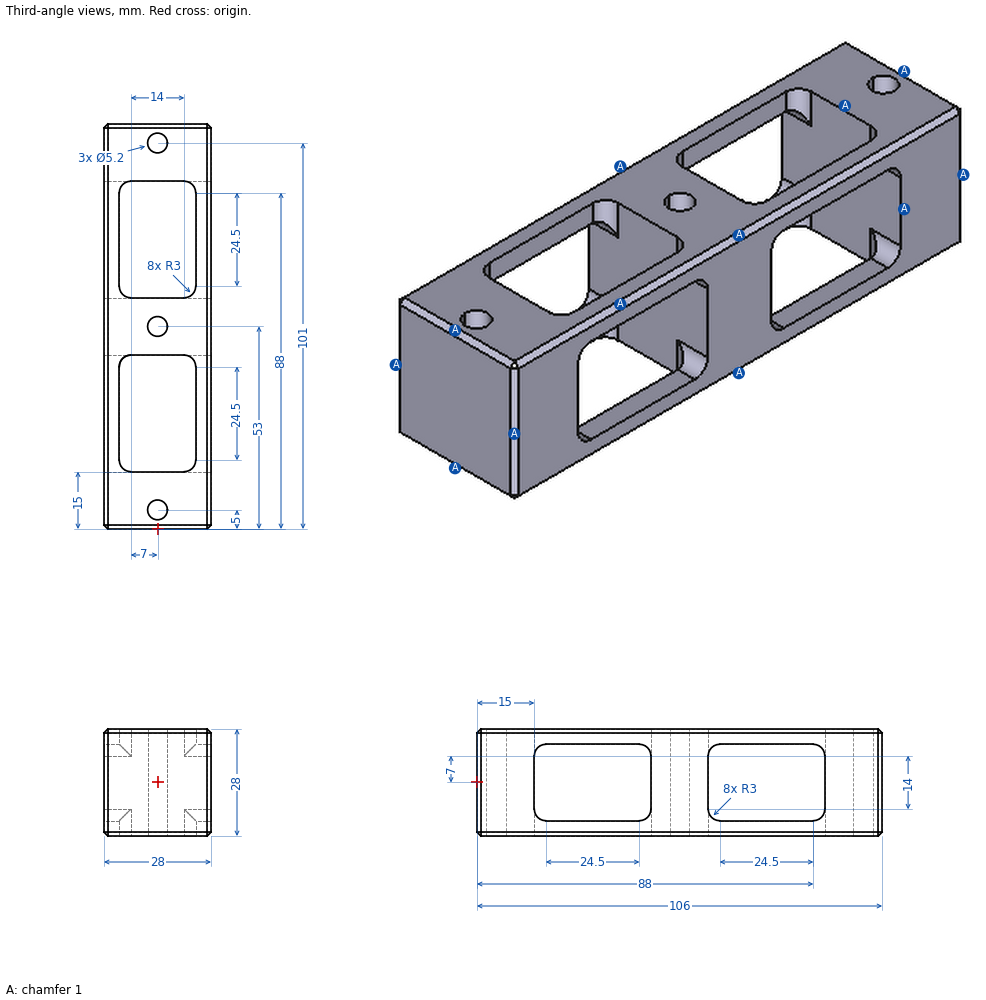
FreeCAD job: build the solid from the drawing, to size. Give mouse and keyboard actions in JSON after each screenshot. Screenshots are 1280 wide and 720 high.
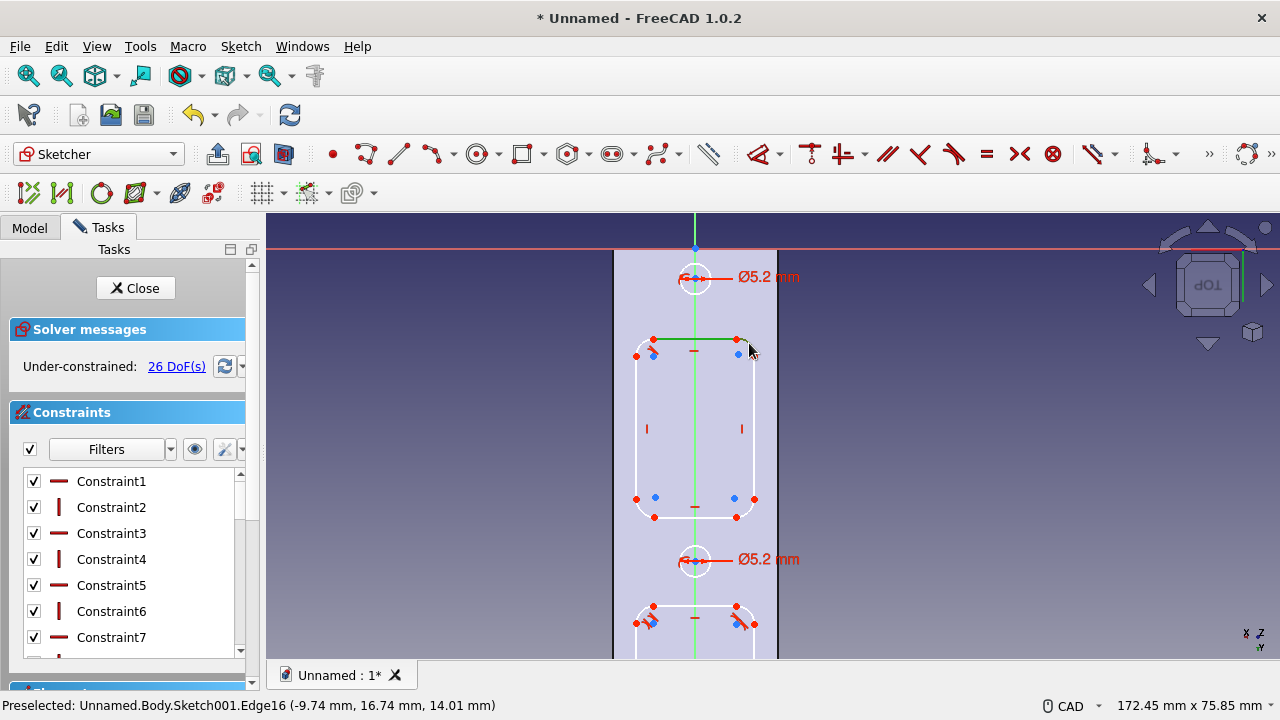
{"action": "left_click", "coordinate": [954, 154]}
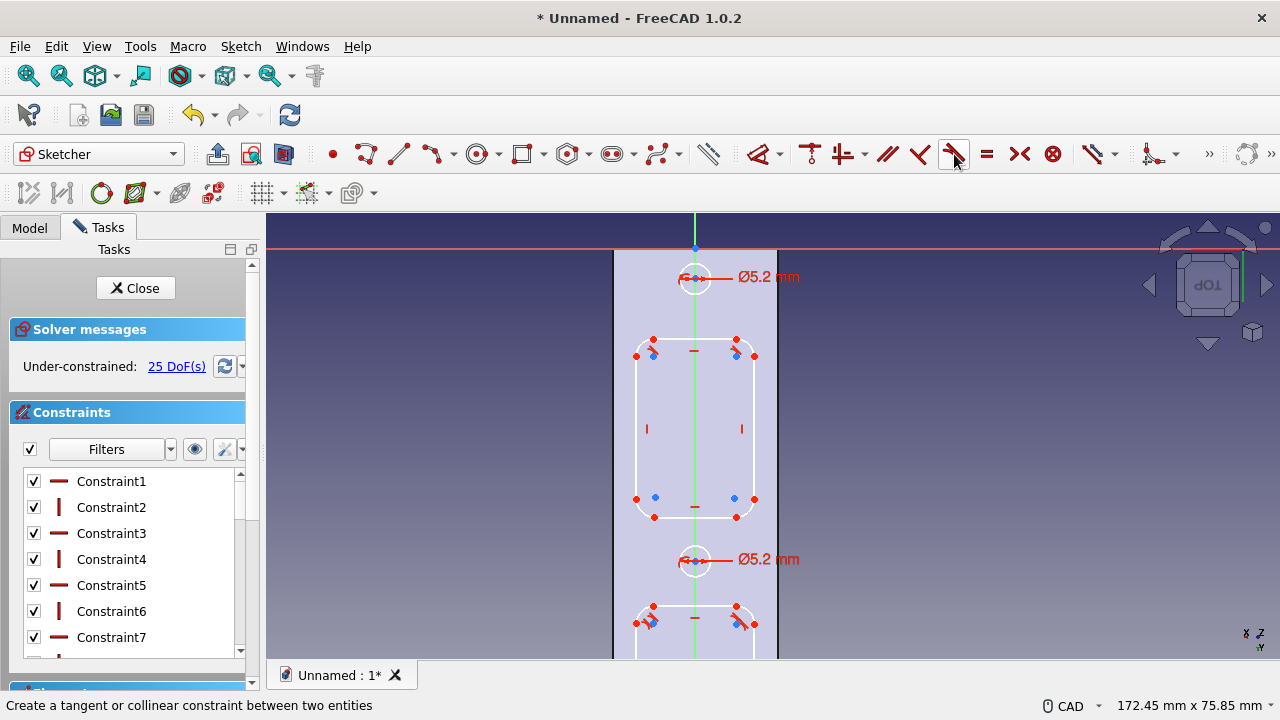
{"action": "left_click", "coordinate": [636, 399]}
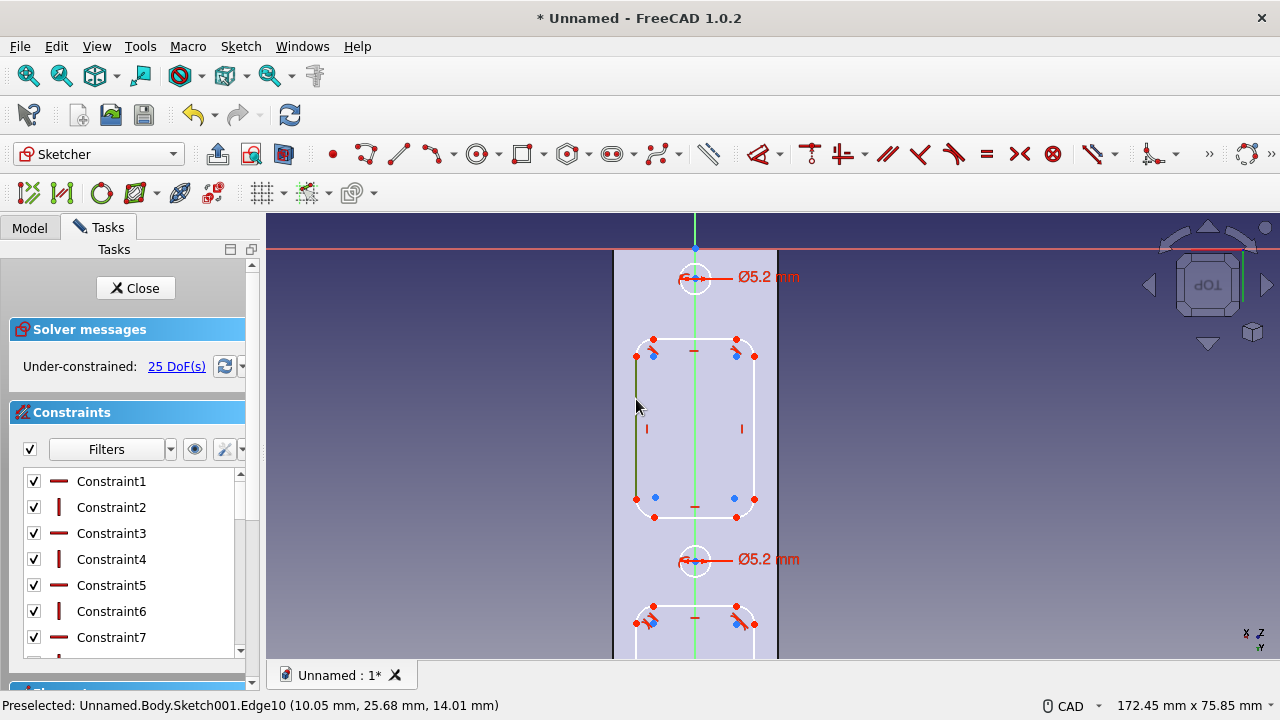
{"action": "left_click", "coordinate": [641, 344]}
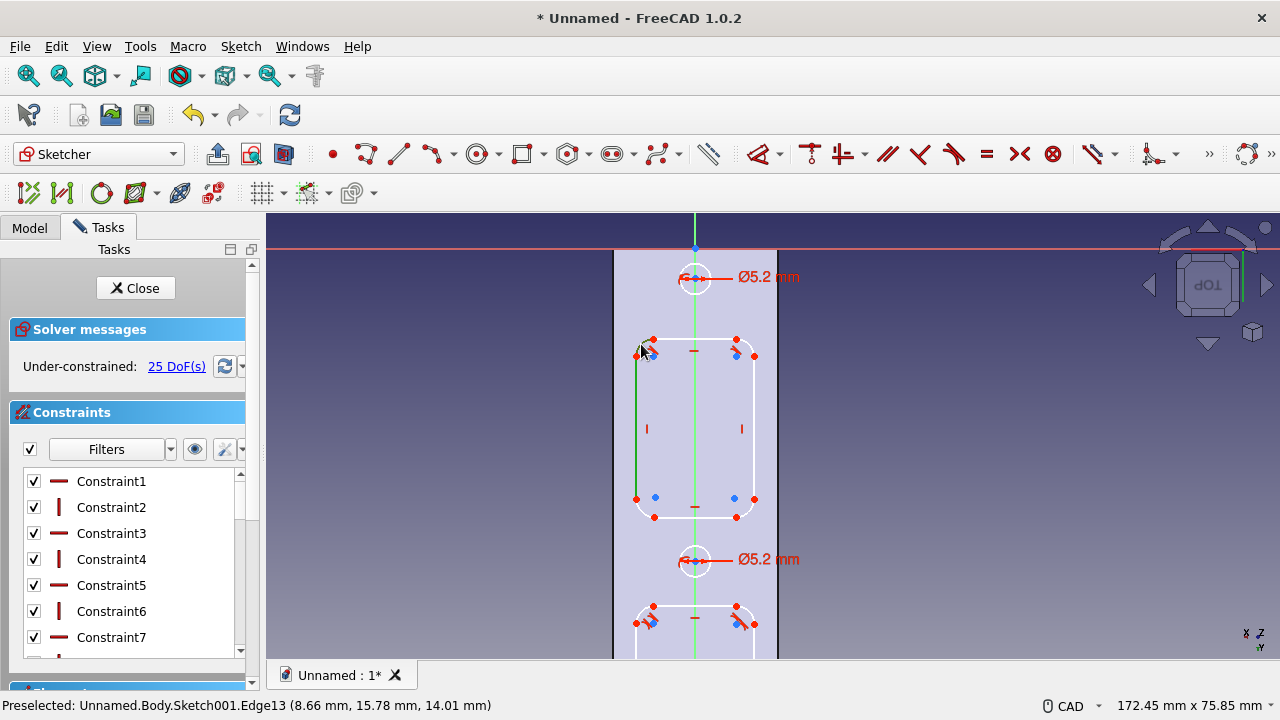
{"action": "key", "text": "t"}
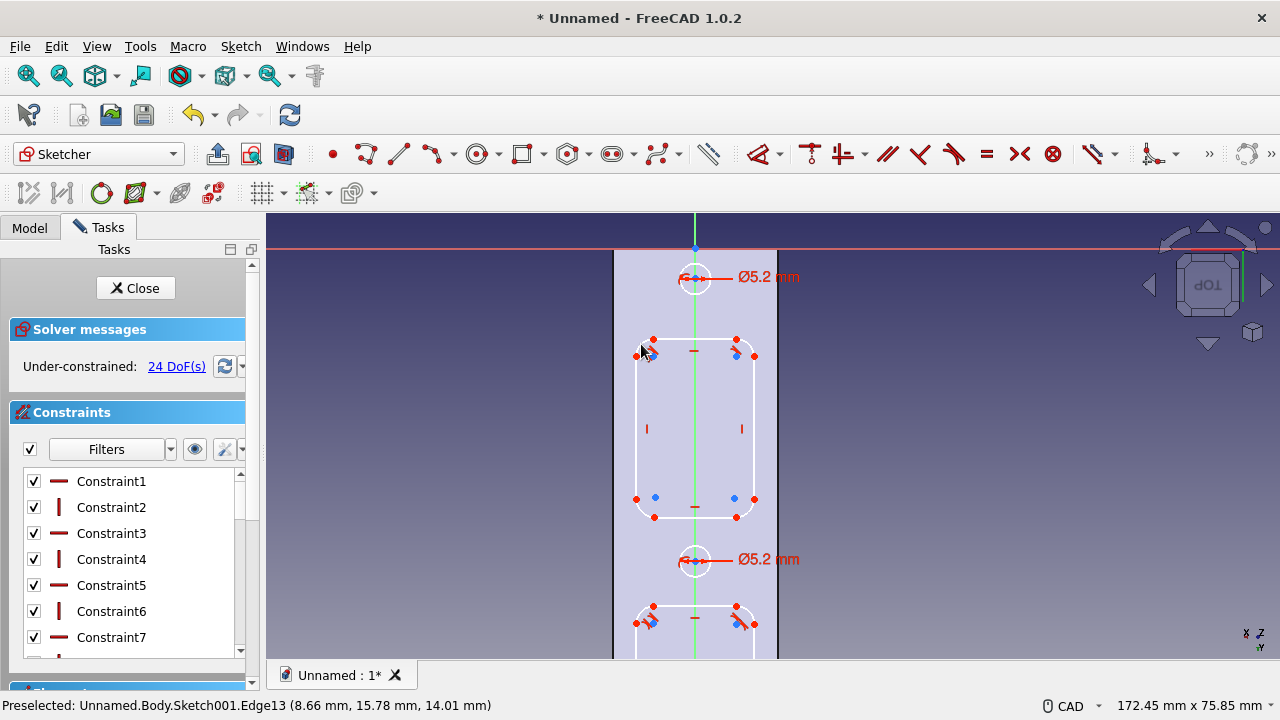
{"action": "left_click", "coordinate": [636, 400]}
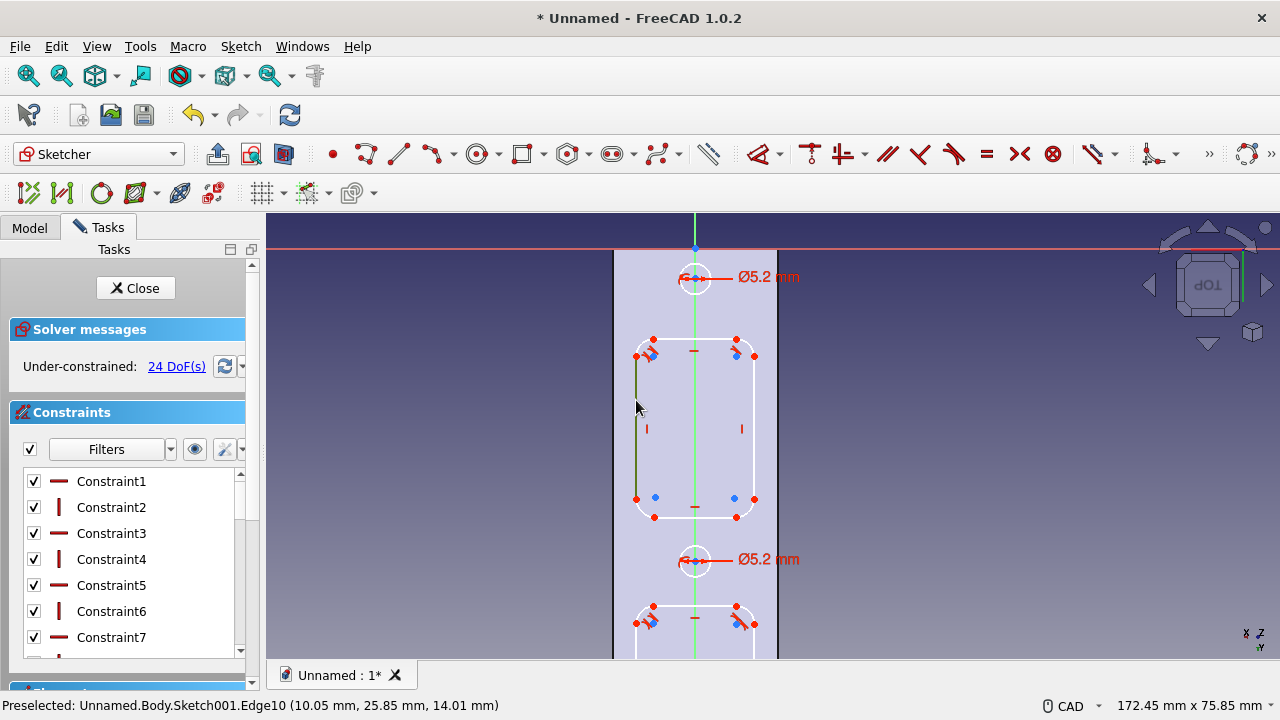
{"action": "left_click", "coordinate": [642, 512]}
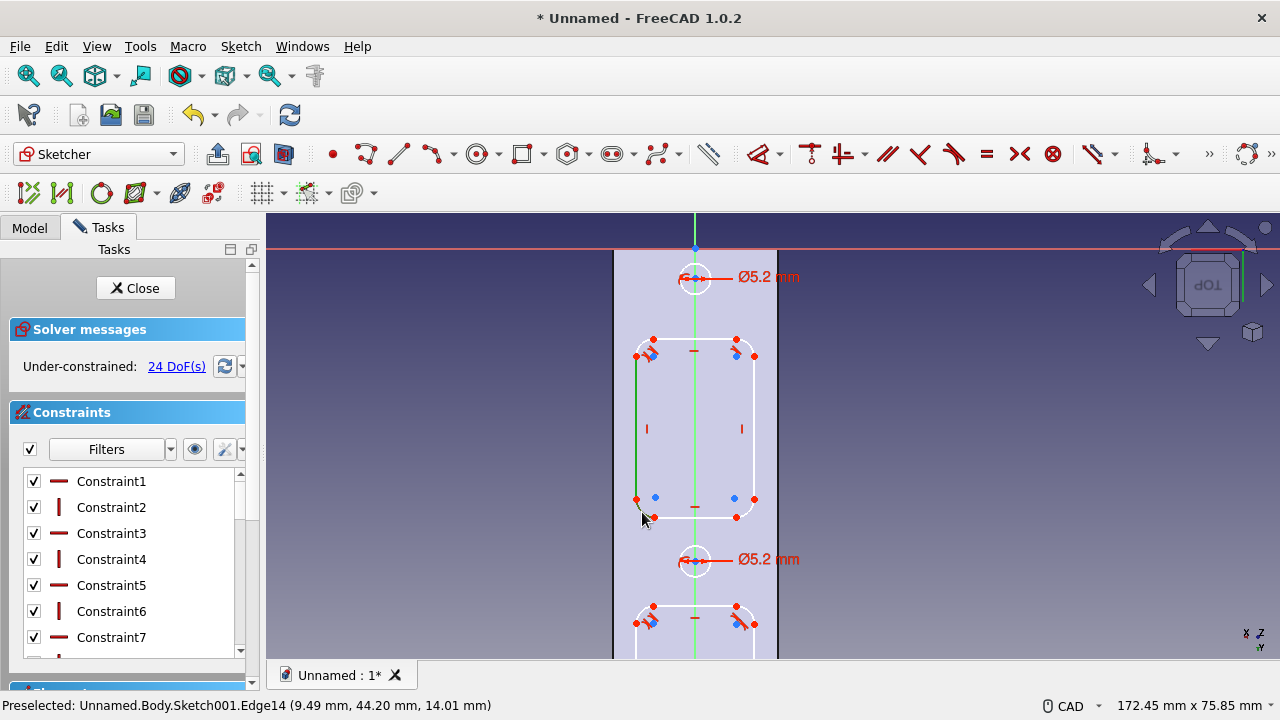
{"action": "left_click", "coordinate": [954, 154]}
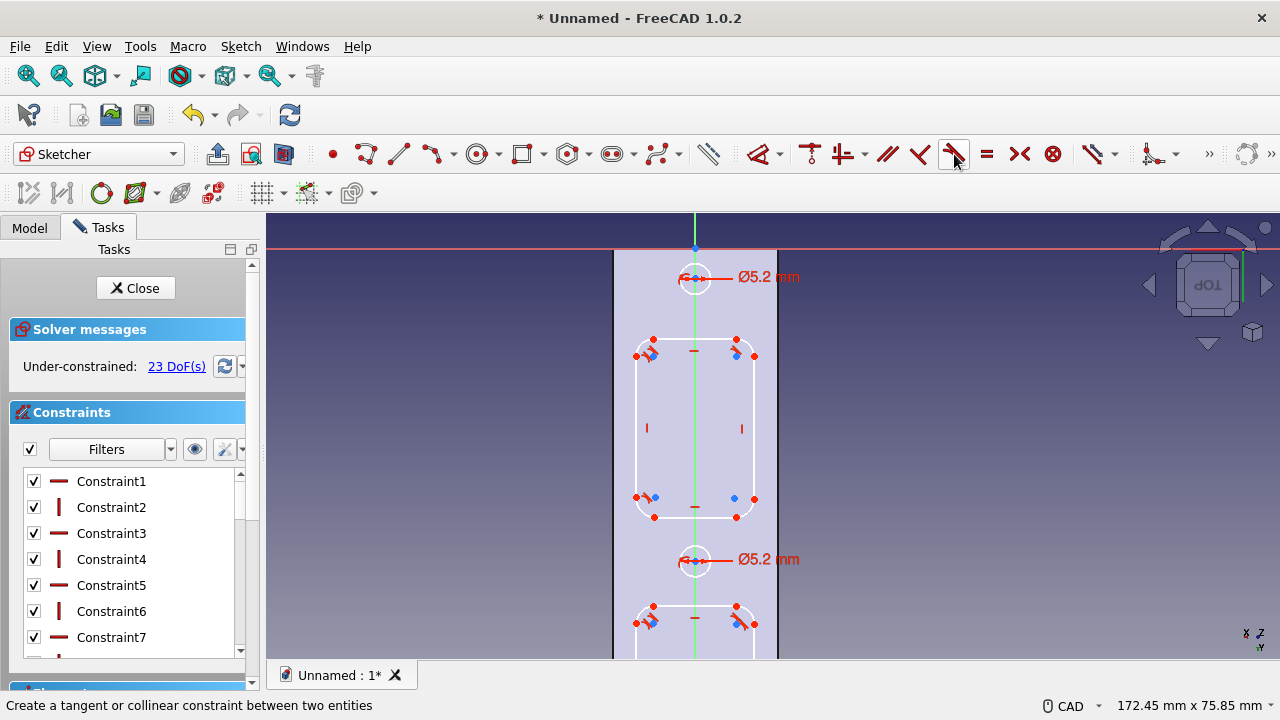
{"action": "left_click", "coordinate": [679, 518]}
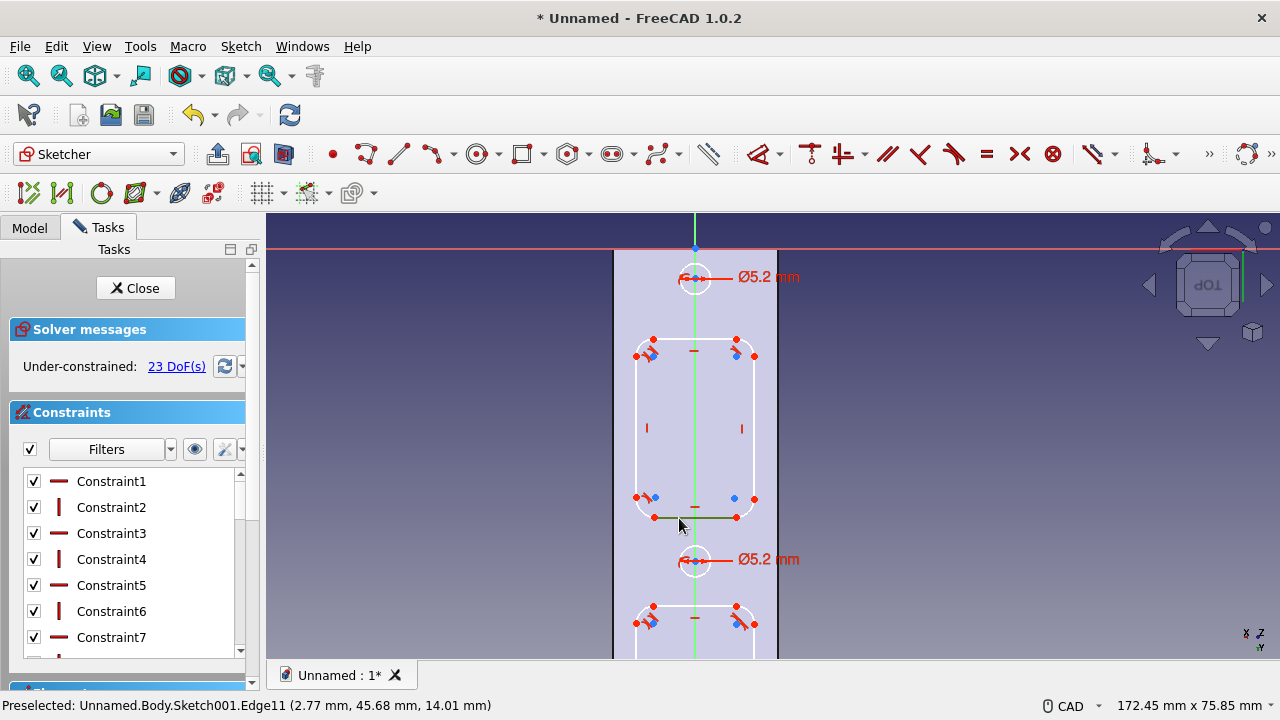
{"action": "left_click", "coordinate": [641, 511]}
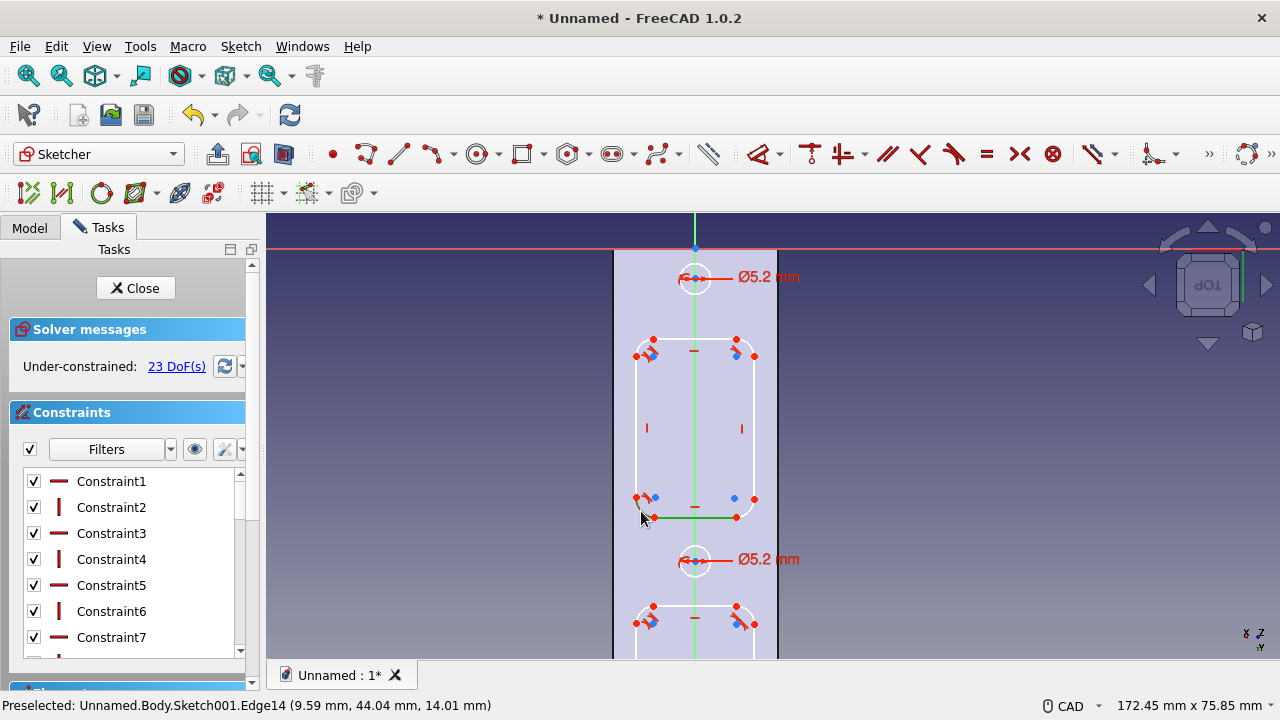
{"action": "left_click", "coordinate": [954, 154]}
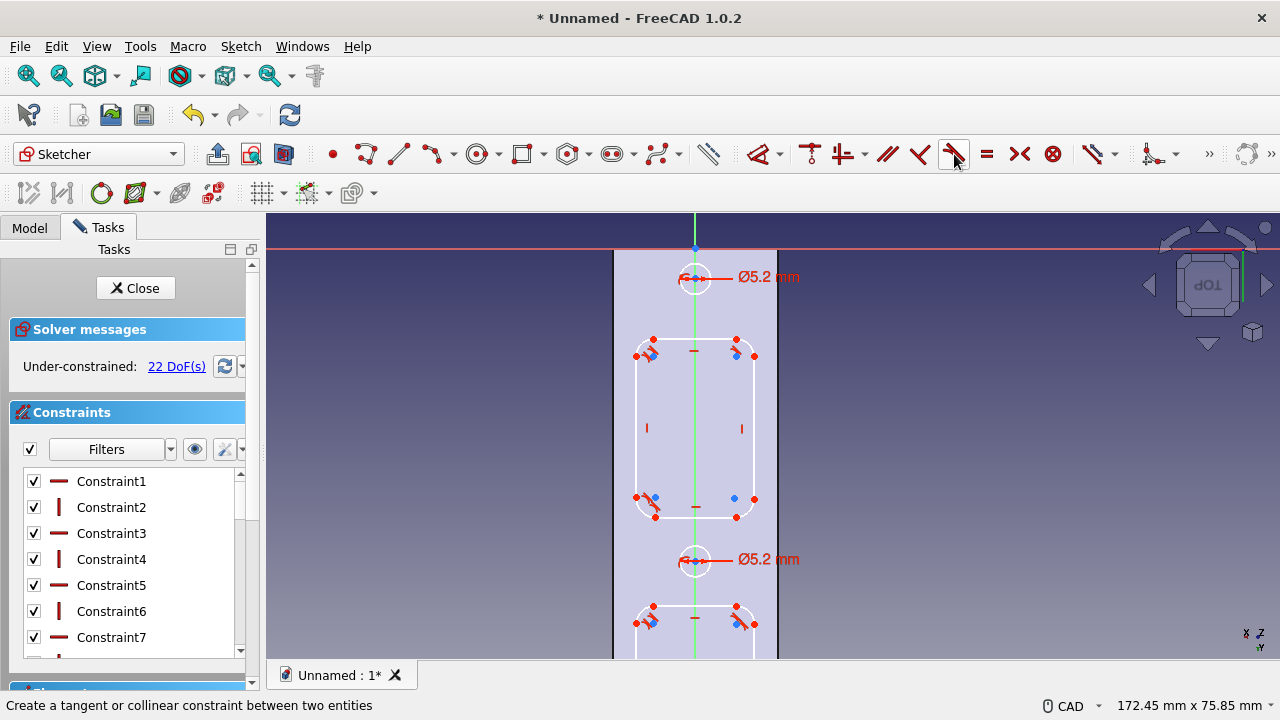
{"action": "left_click", "coordinate": [680, 518]}